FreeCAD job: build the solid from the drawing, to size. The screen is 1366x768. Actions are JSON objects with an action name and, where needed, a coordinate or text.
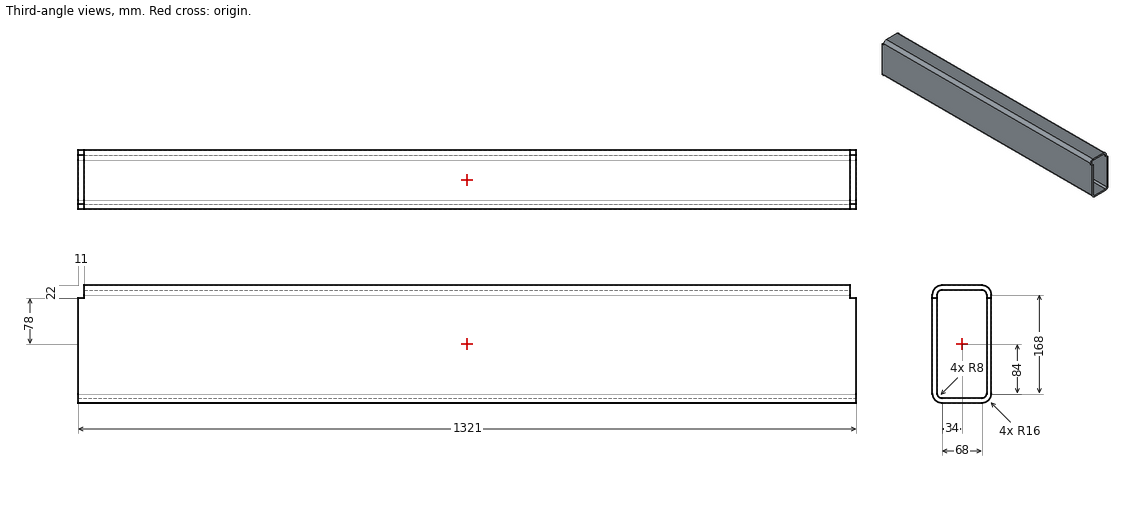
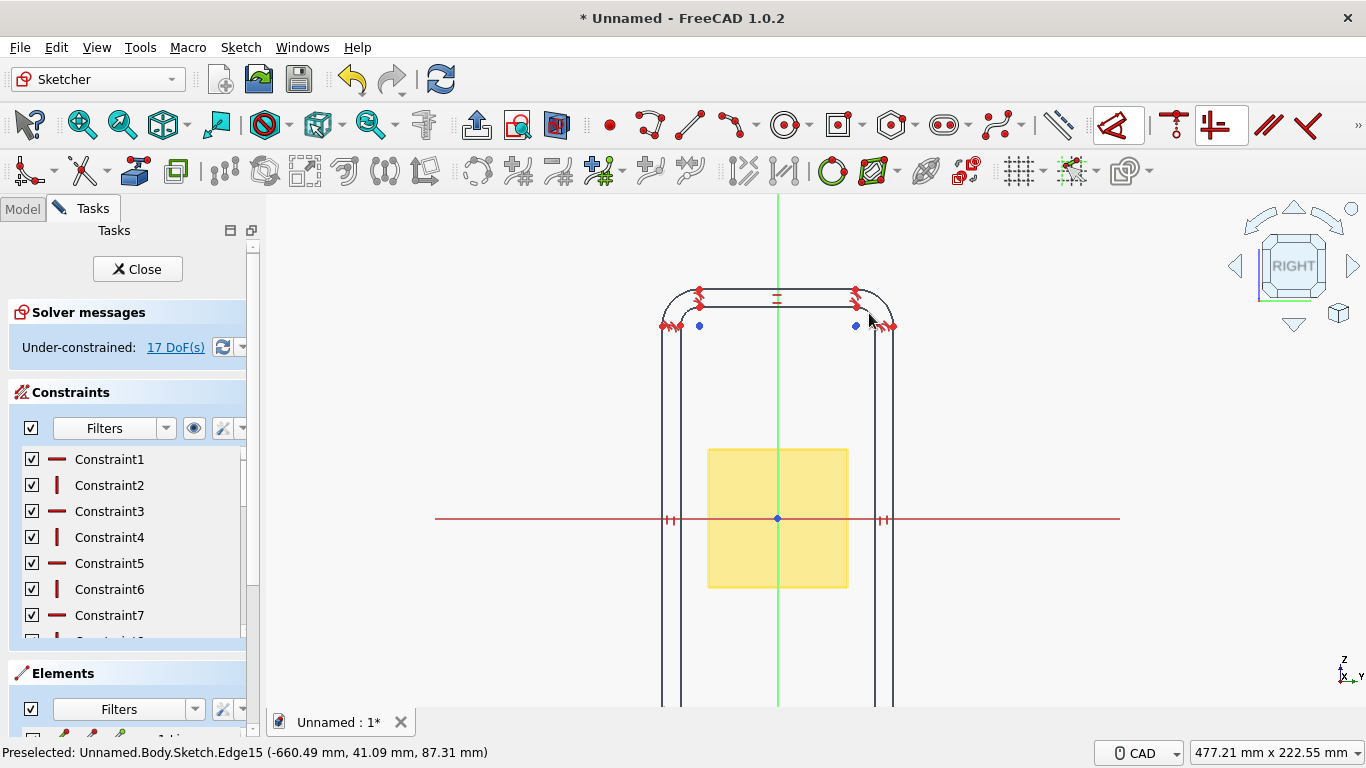
{"action": "left_click", "coordinate": [875, 442]}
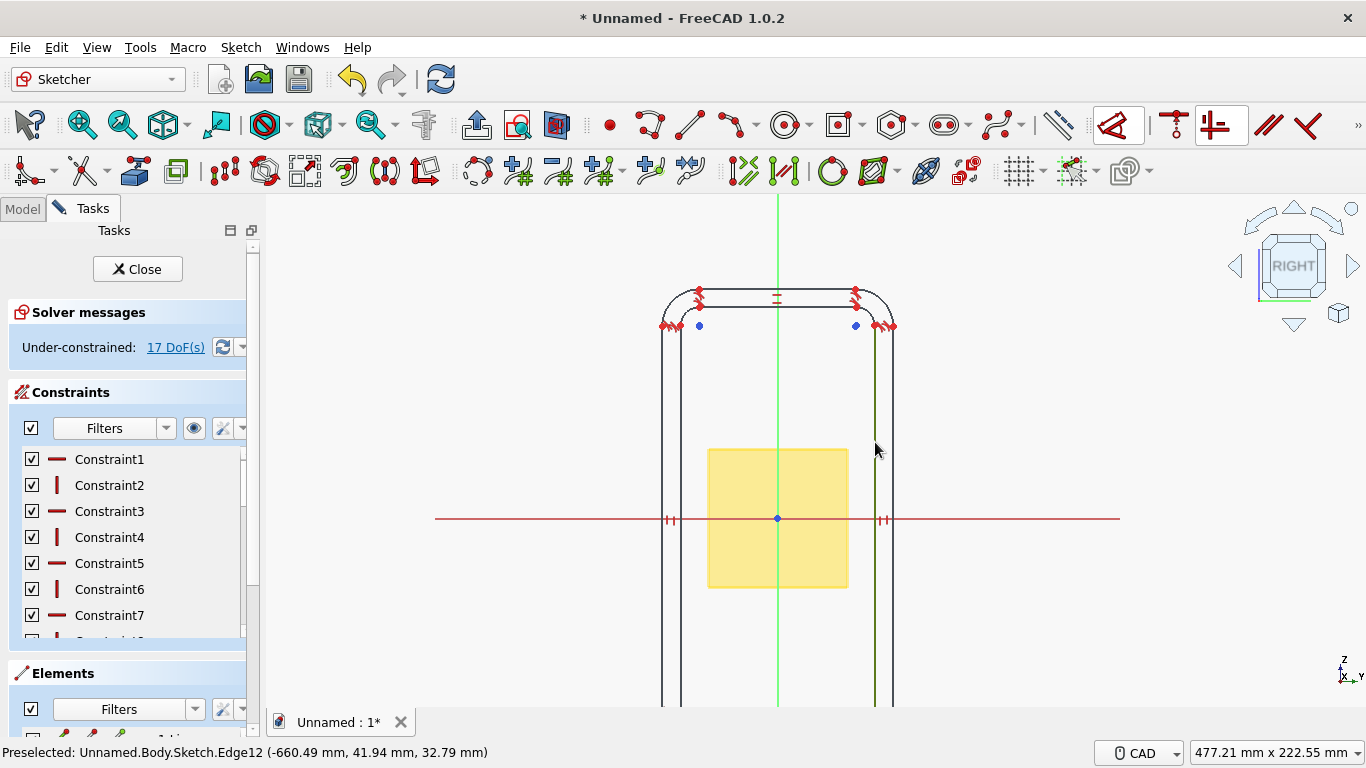
{"action": "scroll", "coordinate": [686, 312], "scroll_direction": "down", "scroll_amount": 2}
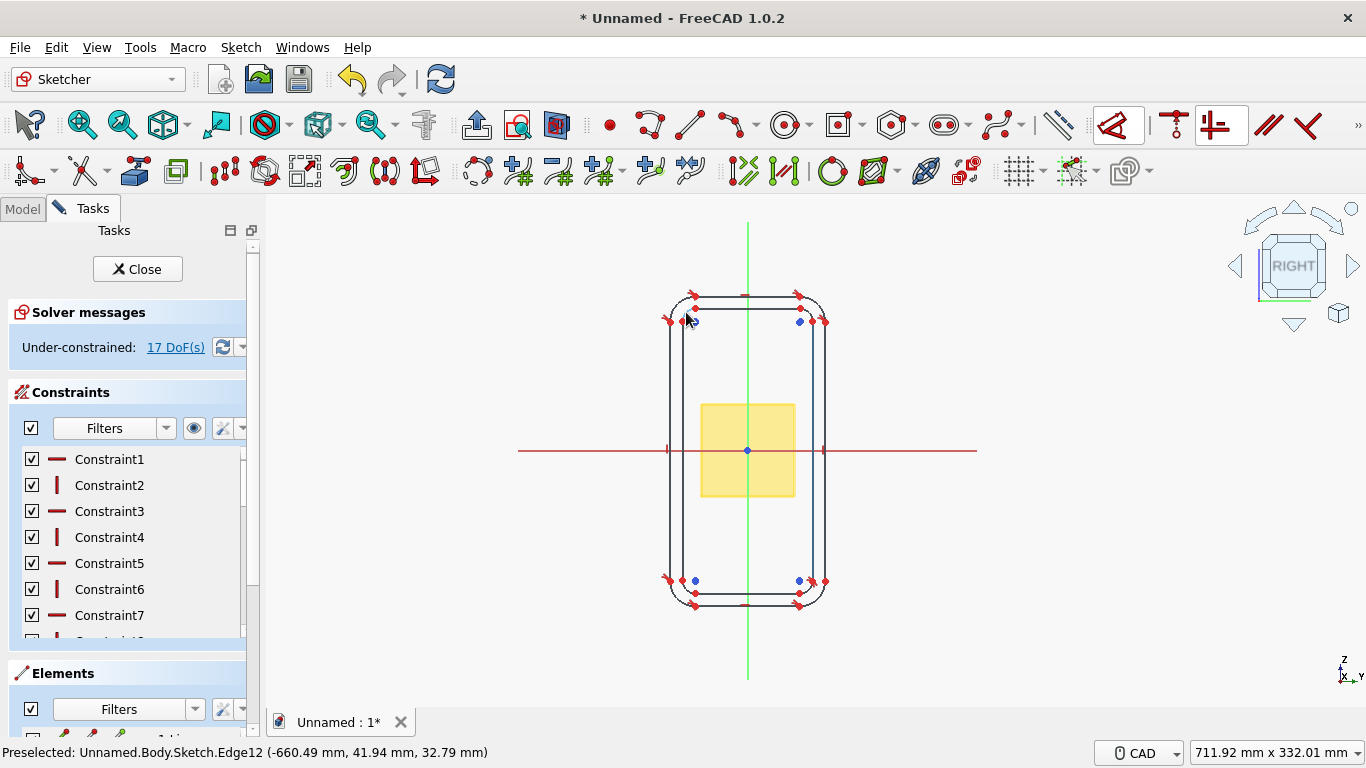
{"action": "scroll", "coordinate": [809, 590], "scroll_direction": "up", "scroll_amount": 2}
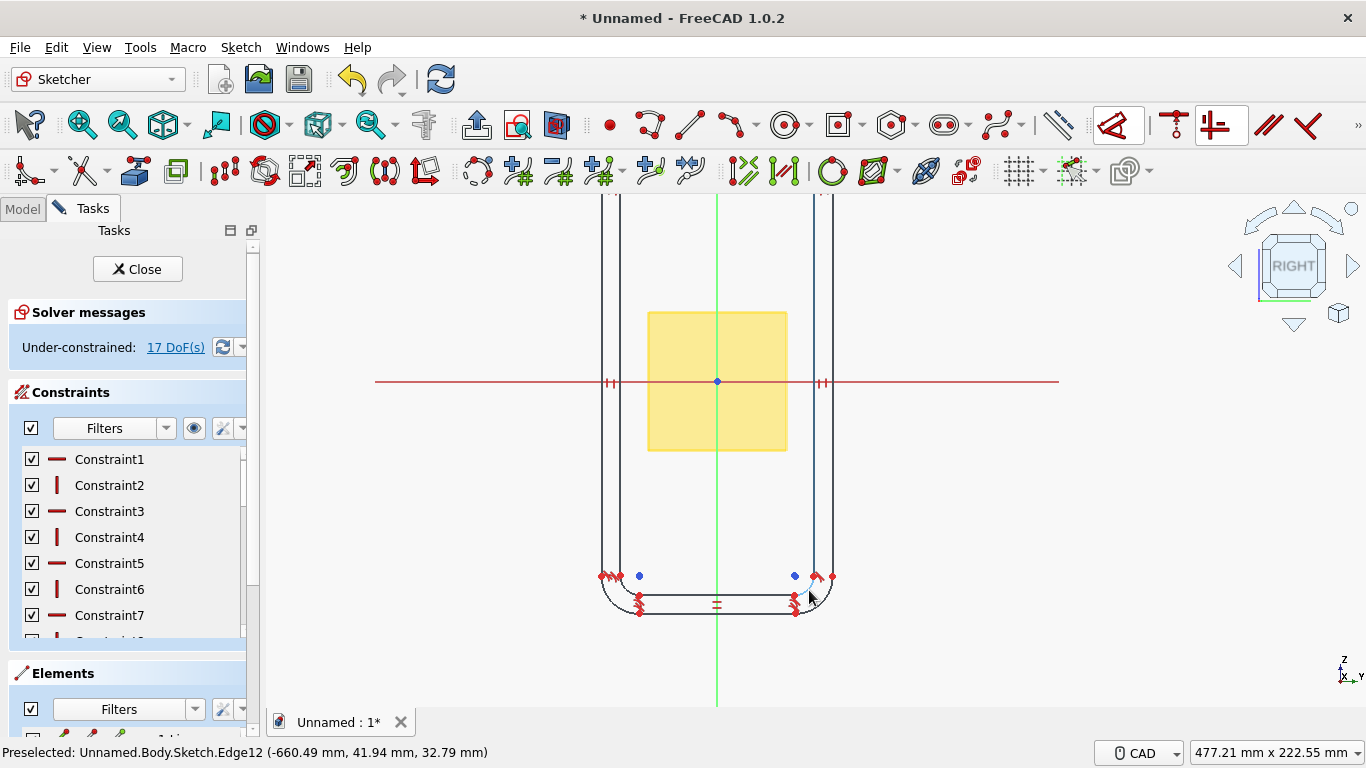
{"action": "left_click", "coordinate": [808, 590]}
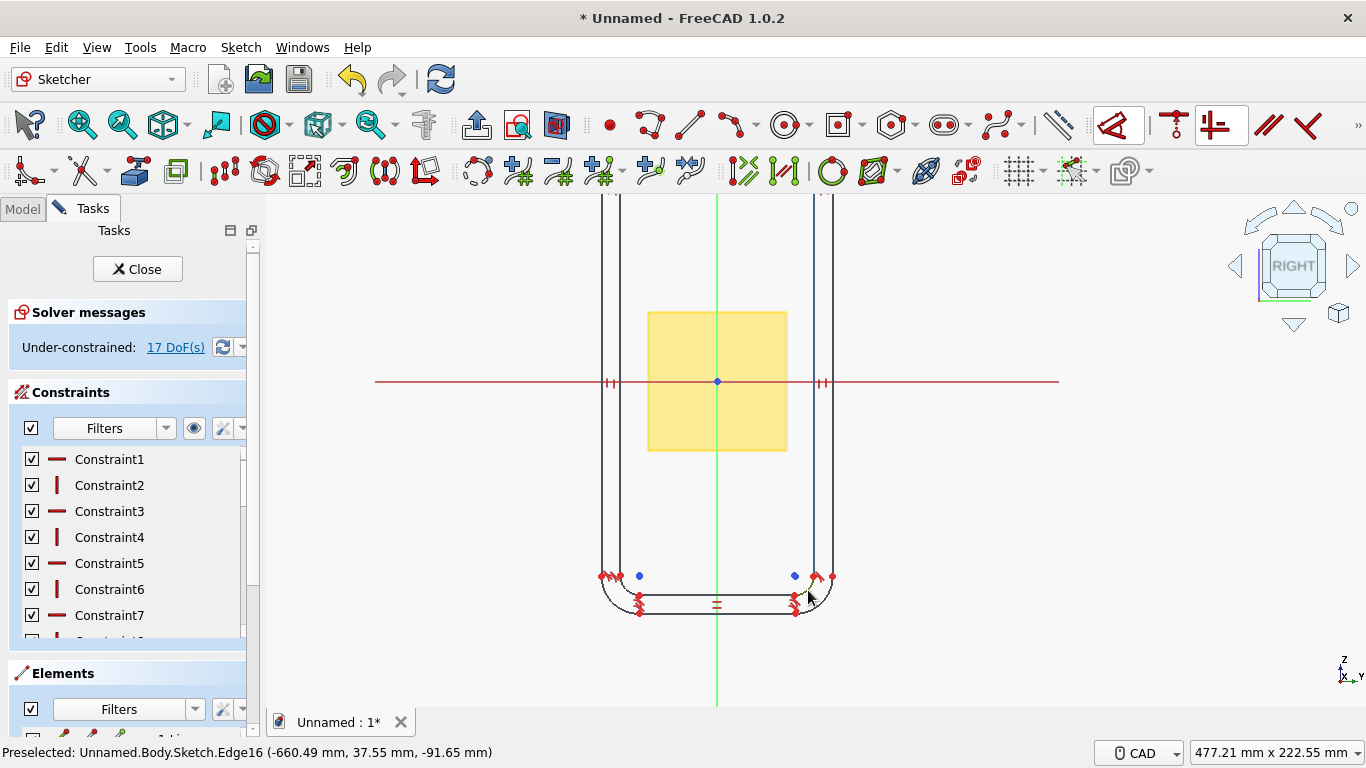
{"action": "key", "text": "t"}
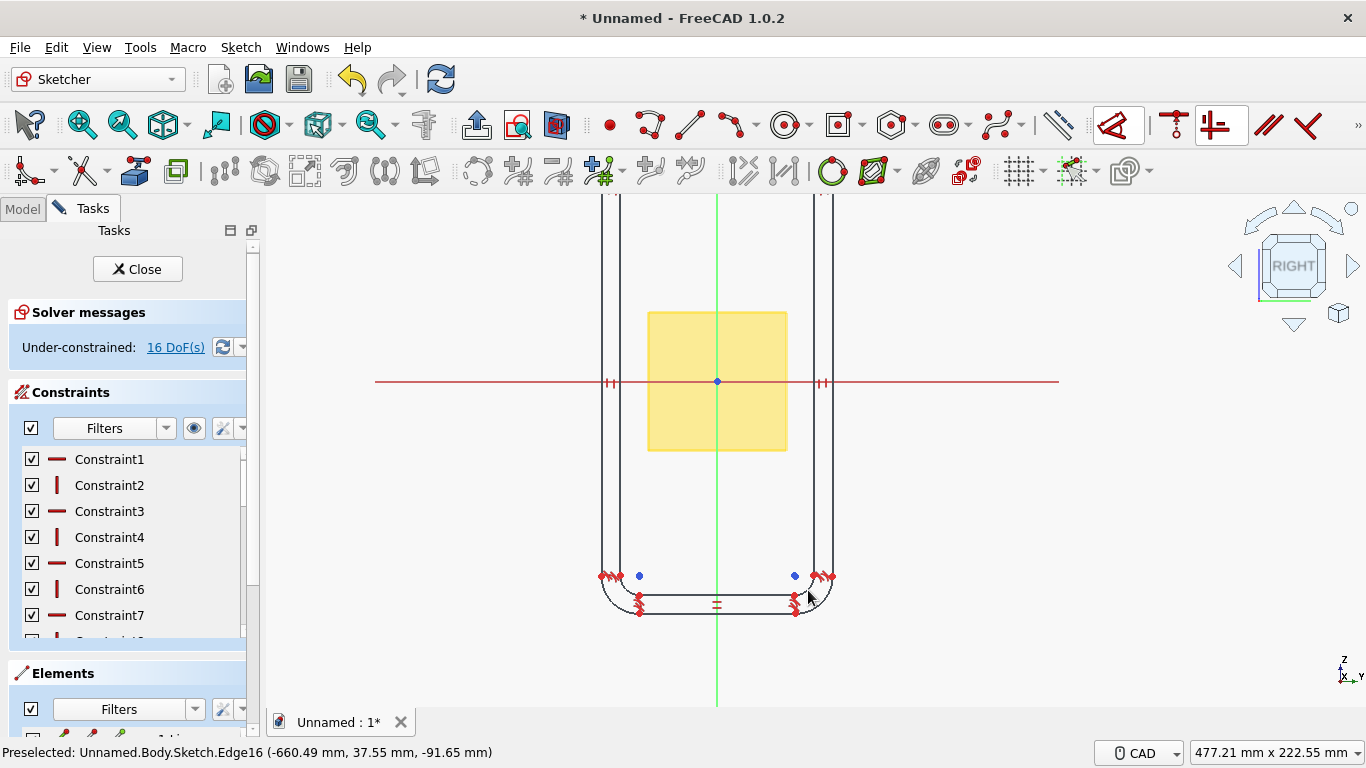
{"action": "left_click", "coordinate": [606, 593]}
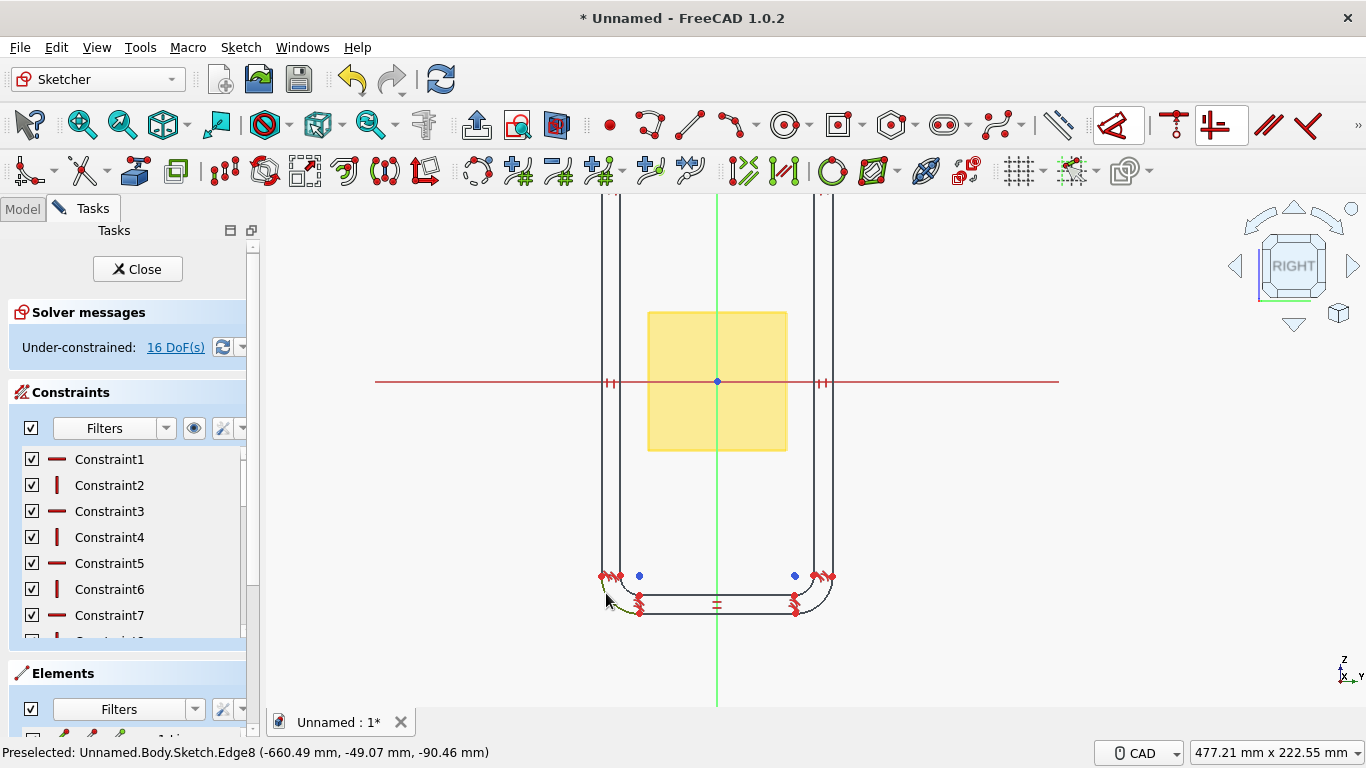
{"action": "scroll", "coordinate": [622, 584], "scroll_direction": "up", "scroll_amount": 3}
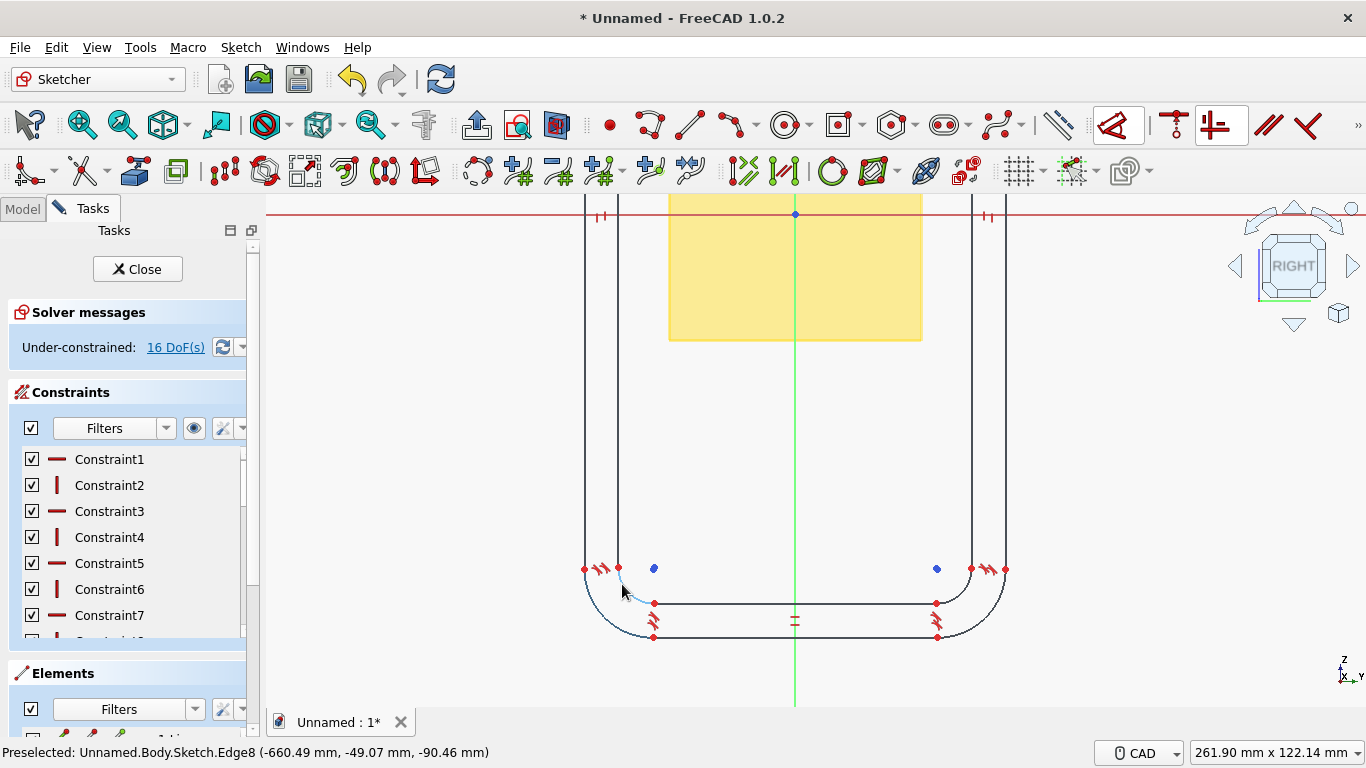
{"action": "left_click", "coordinate": [622, 584]}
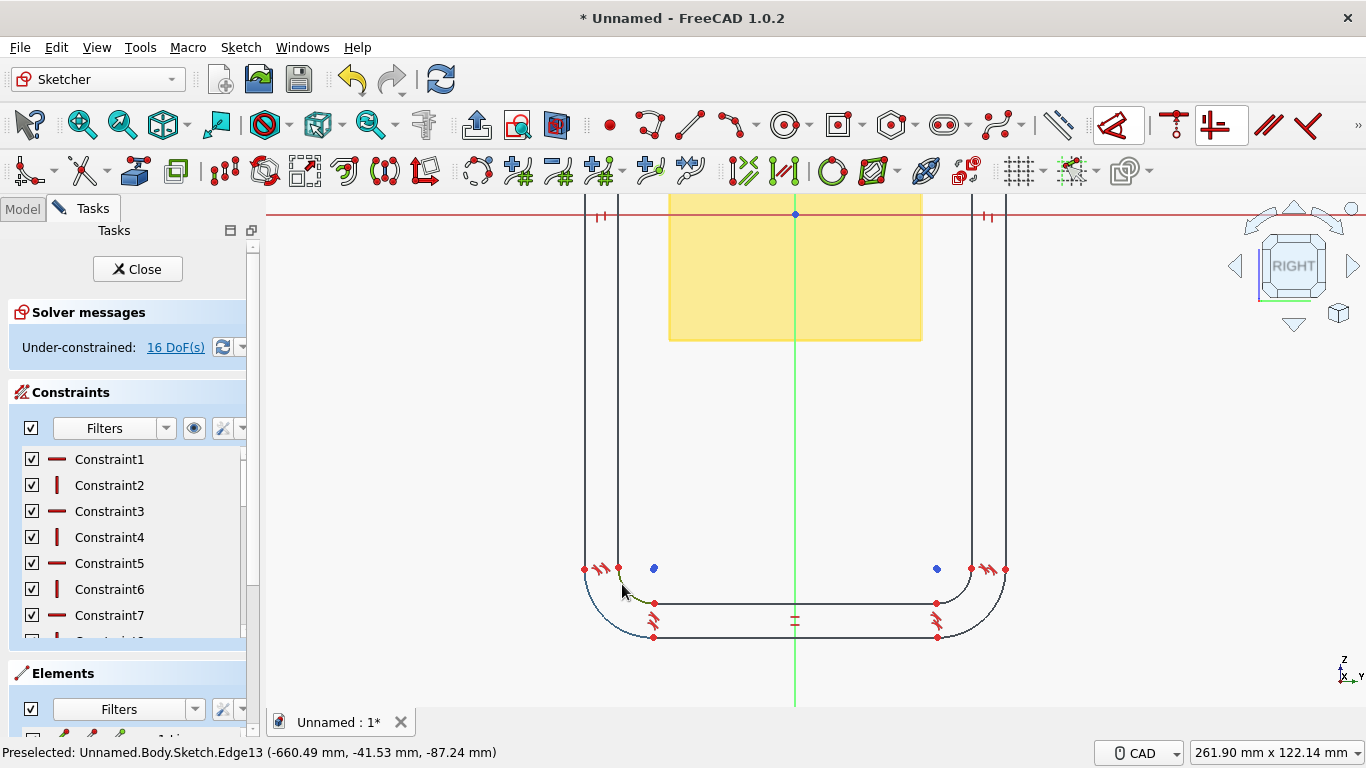
{"action": "left_click", "coordinate": [1174, 126]}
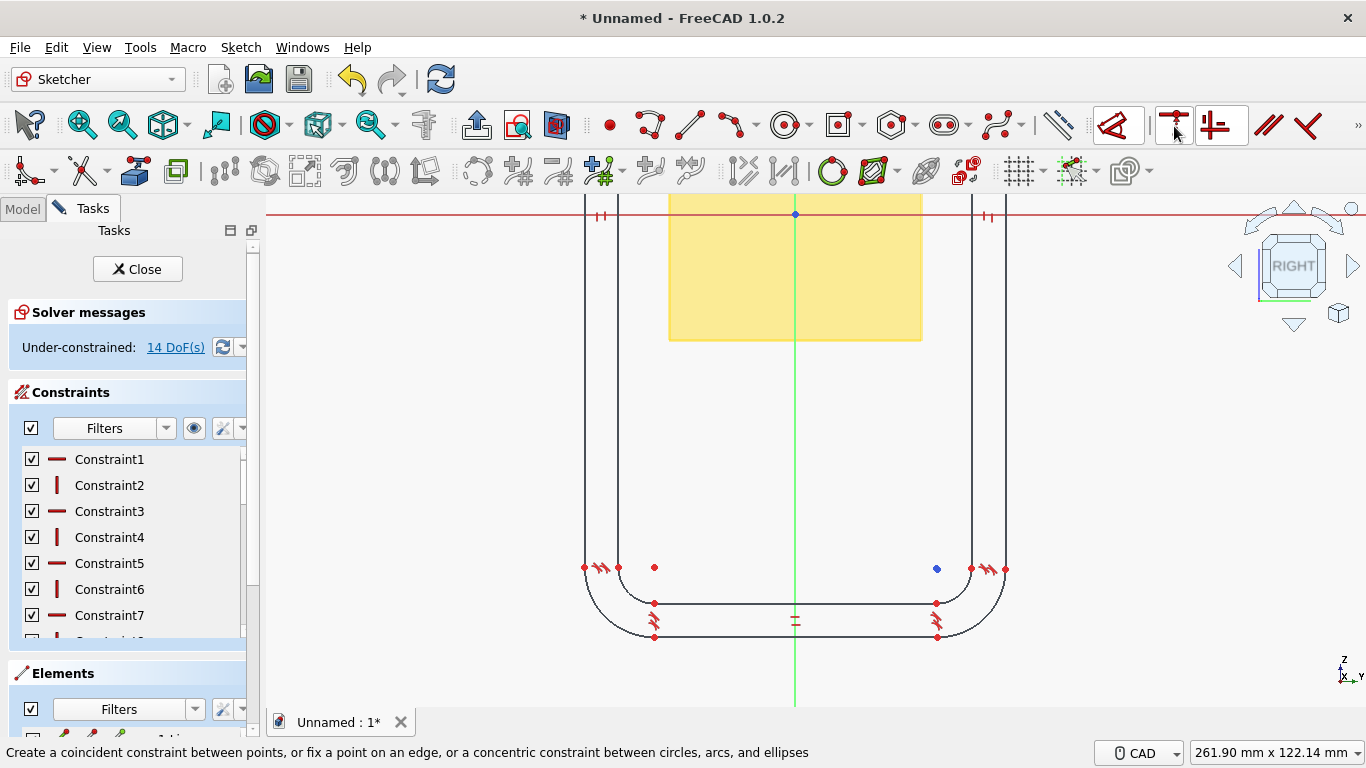
{"action": "scroll", "coordinate": [720, 588], "scroll_direction": "down", "scroll_amount": 5}